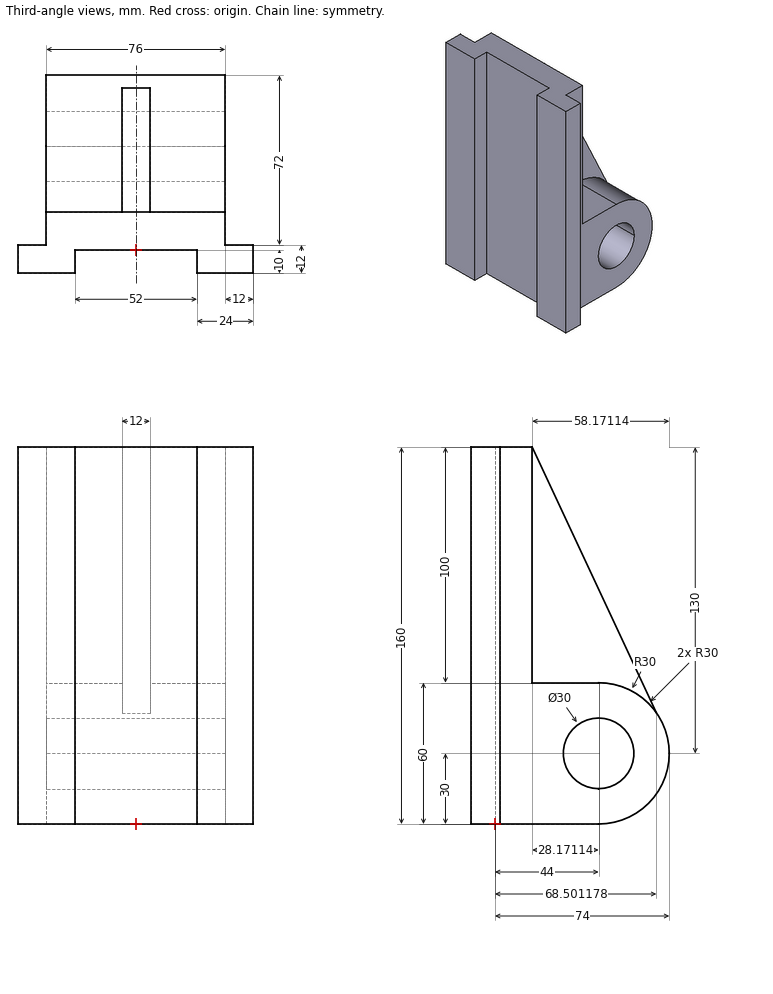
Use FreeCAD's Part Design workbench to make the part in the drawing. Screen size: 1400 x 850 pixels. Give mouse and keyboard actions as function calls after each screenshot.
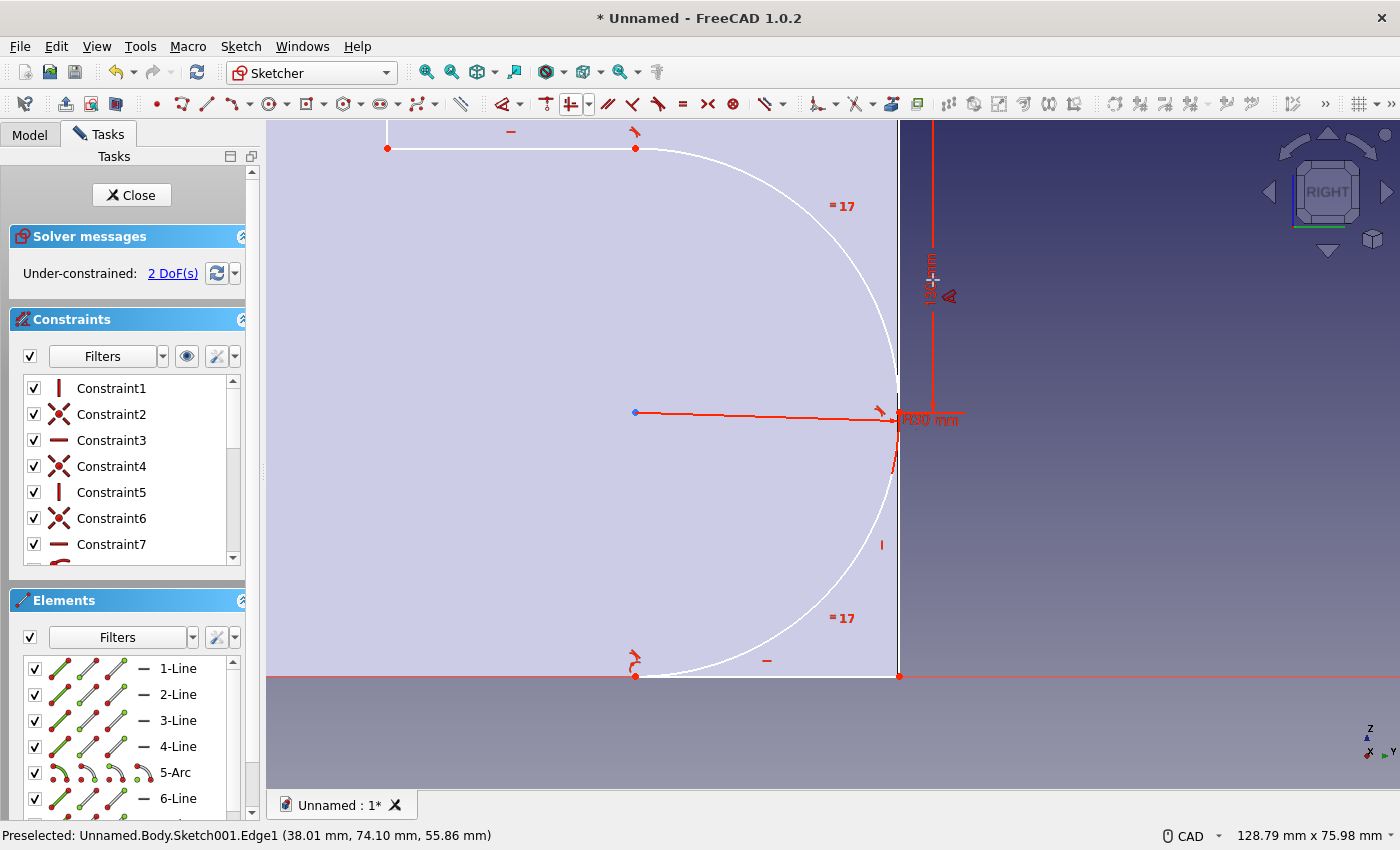
click(899, 413)
click(597, 711)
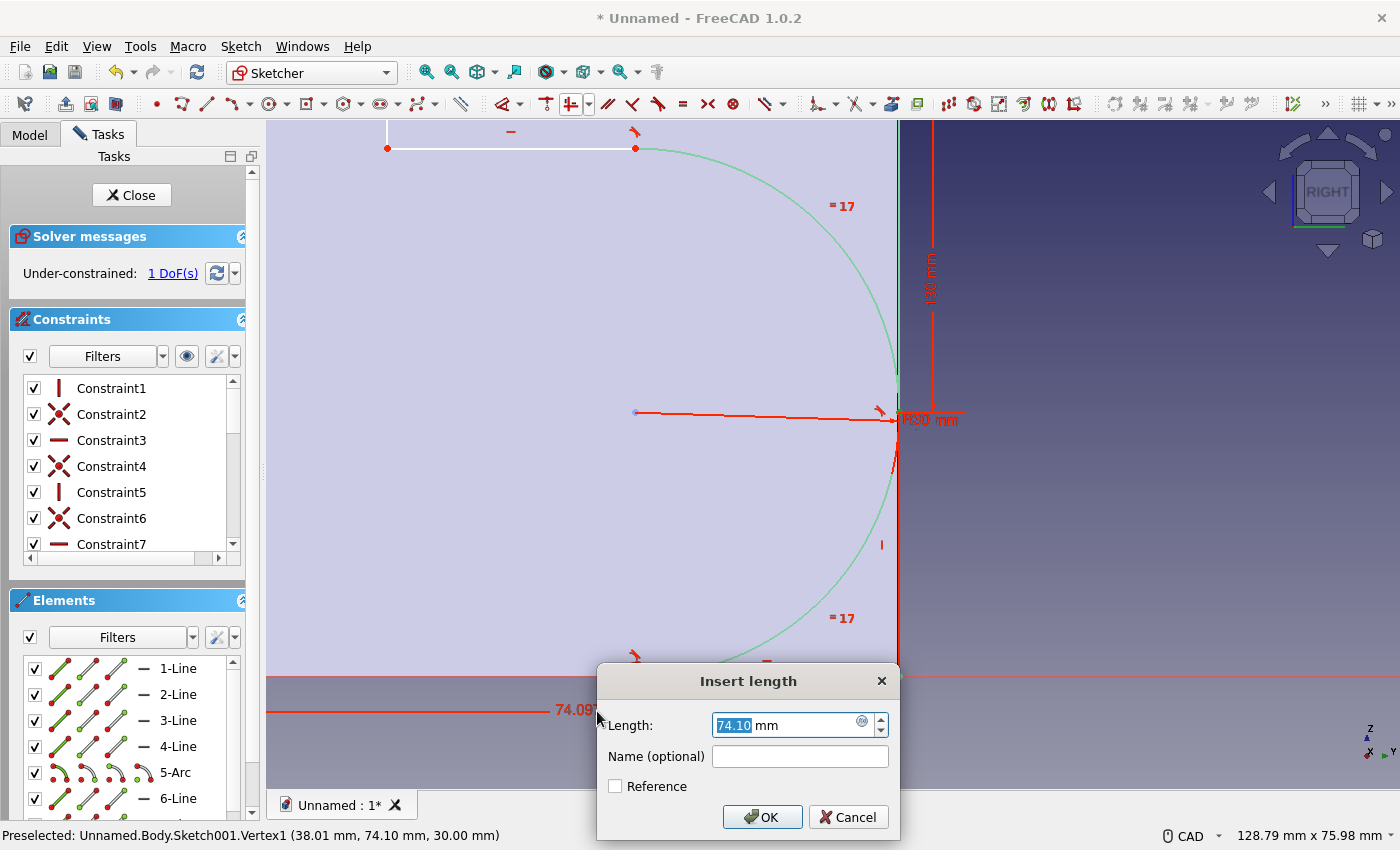
text(74)
key(Return)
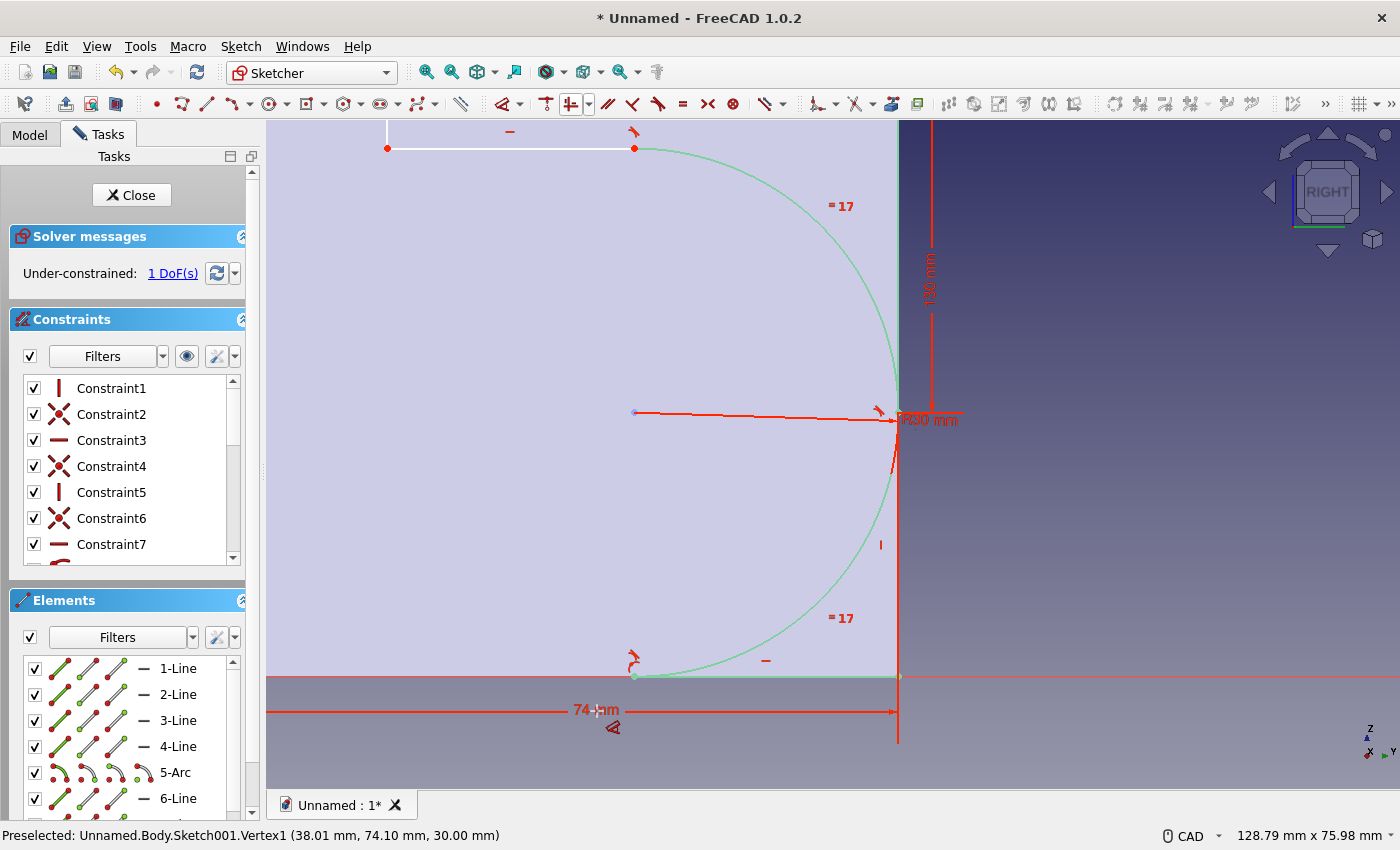
scroll(847, 662, down, 6)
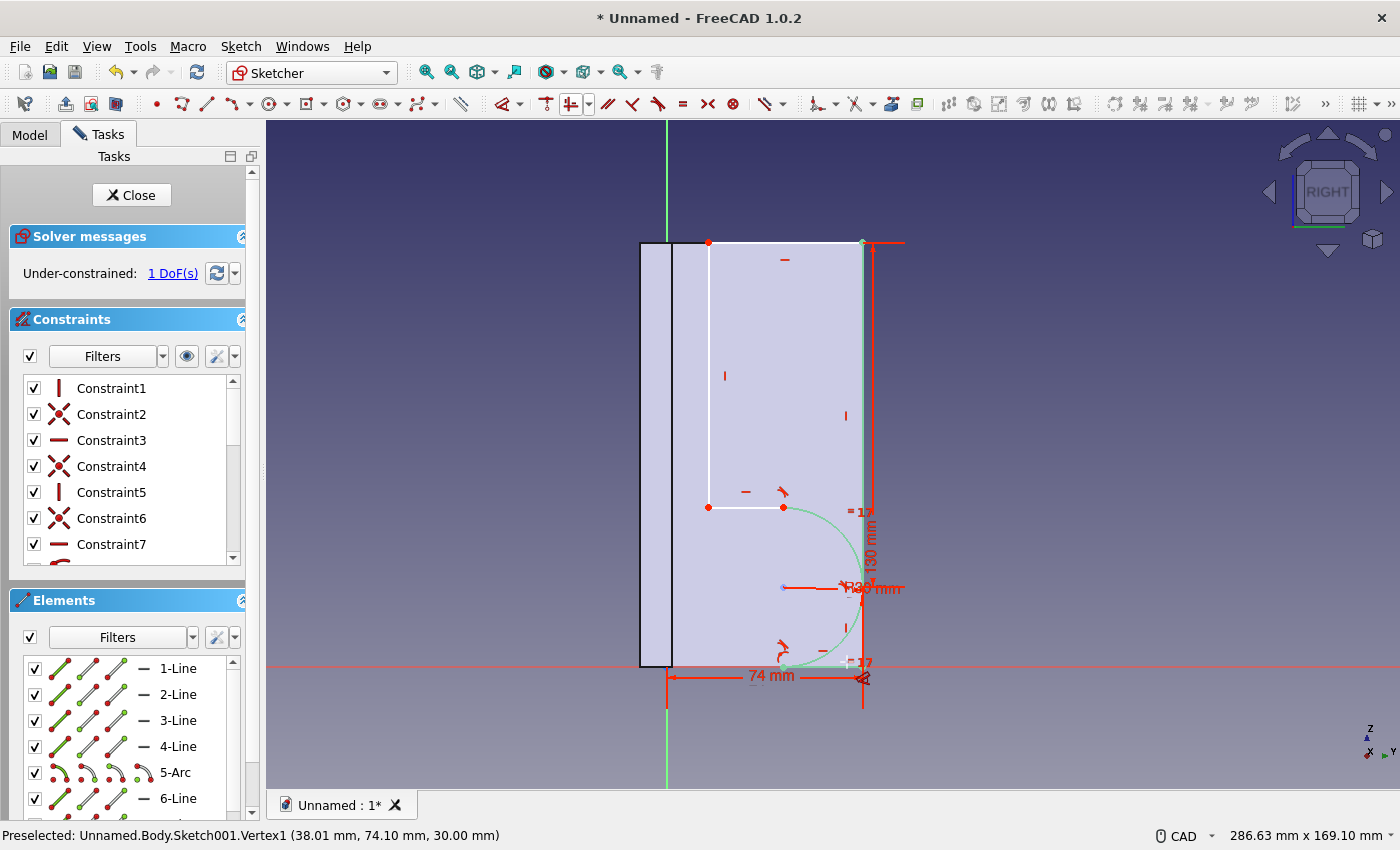
click(817, 243)
click(786, 209)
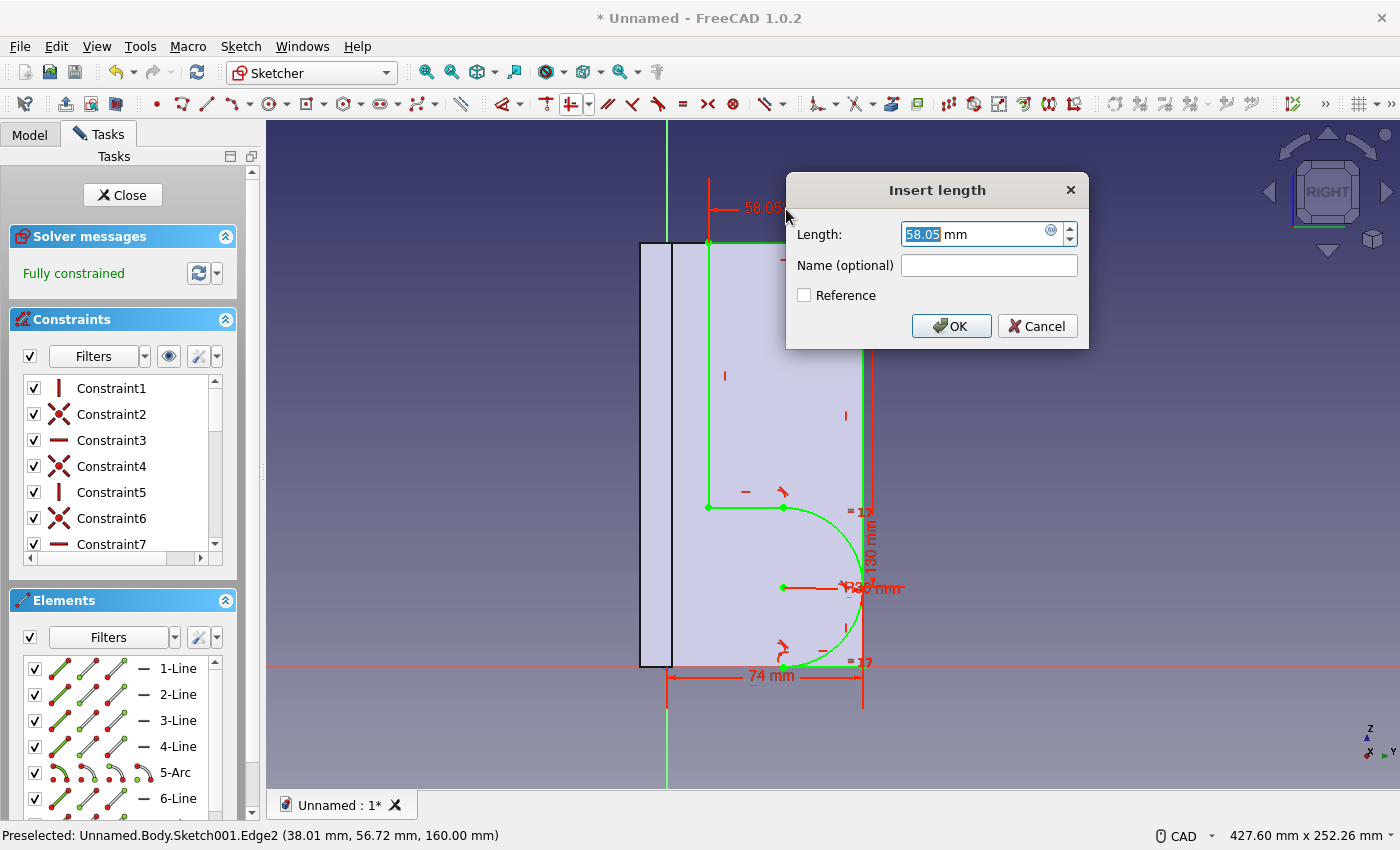
text(58.17114)
key(Return)
key(Escape)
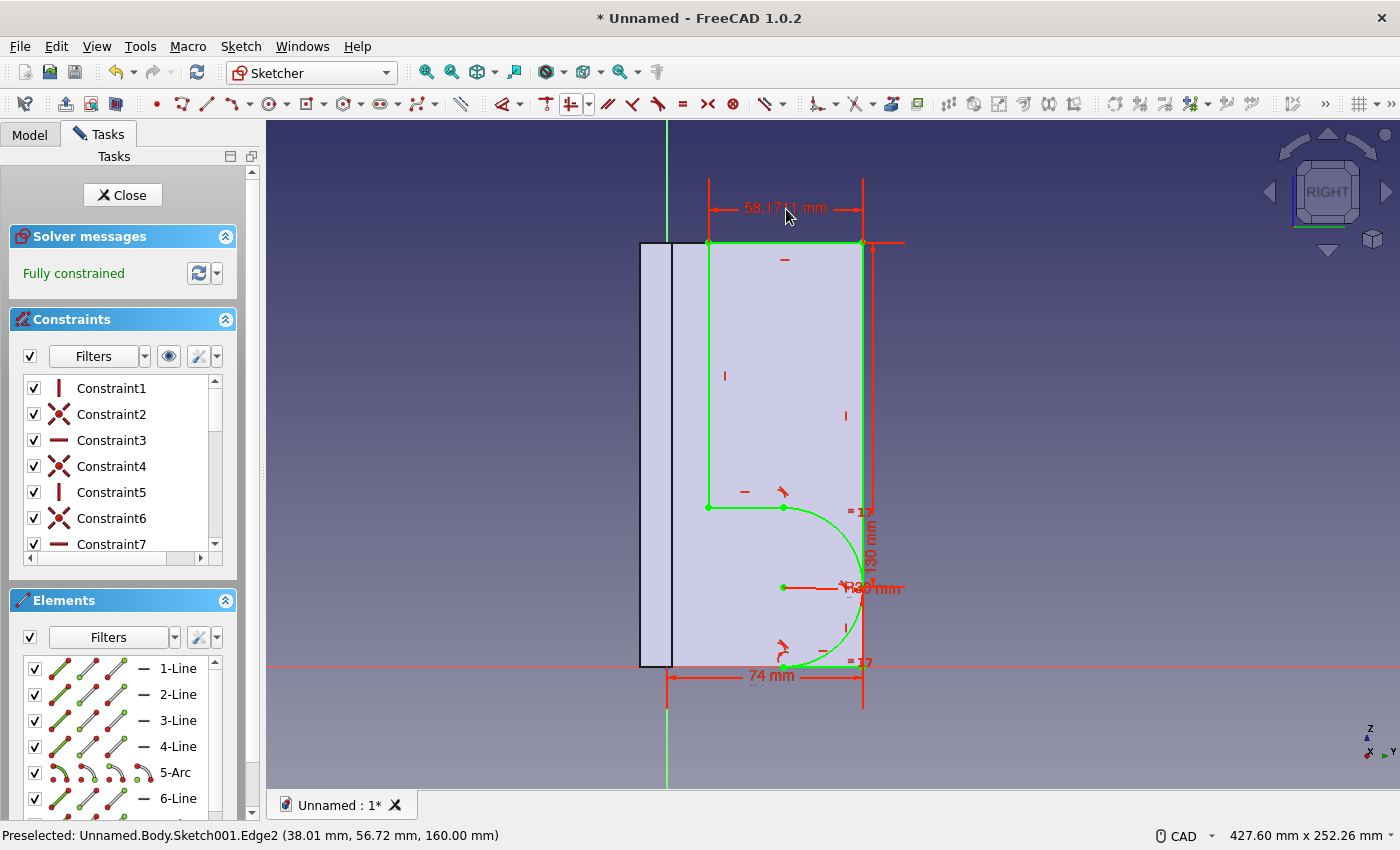
click(123, 195)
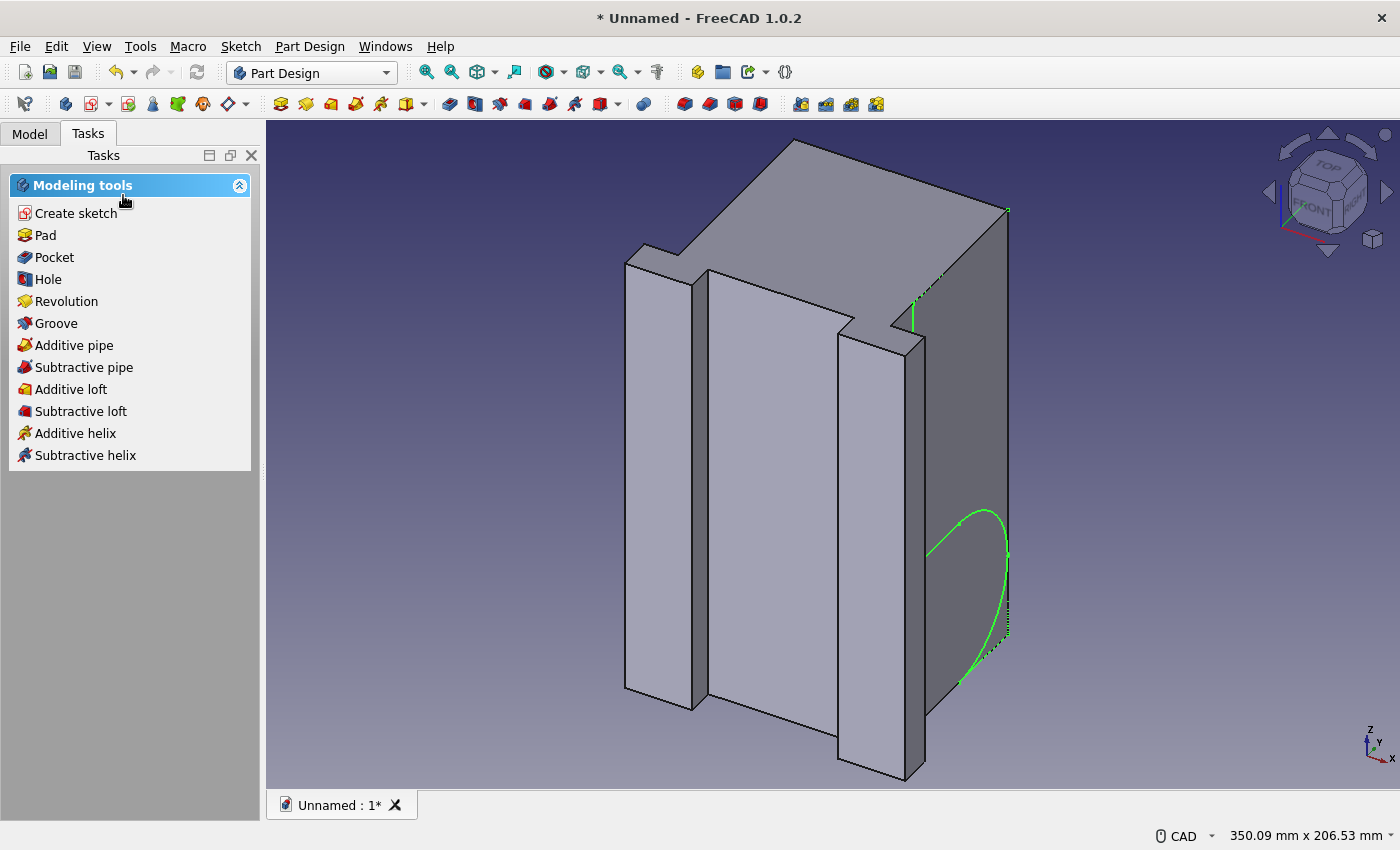
click(450, 104)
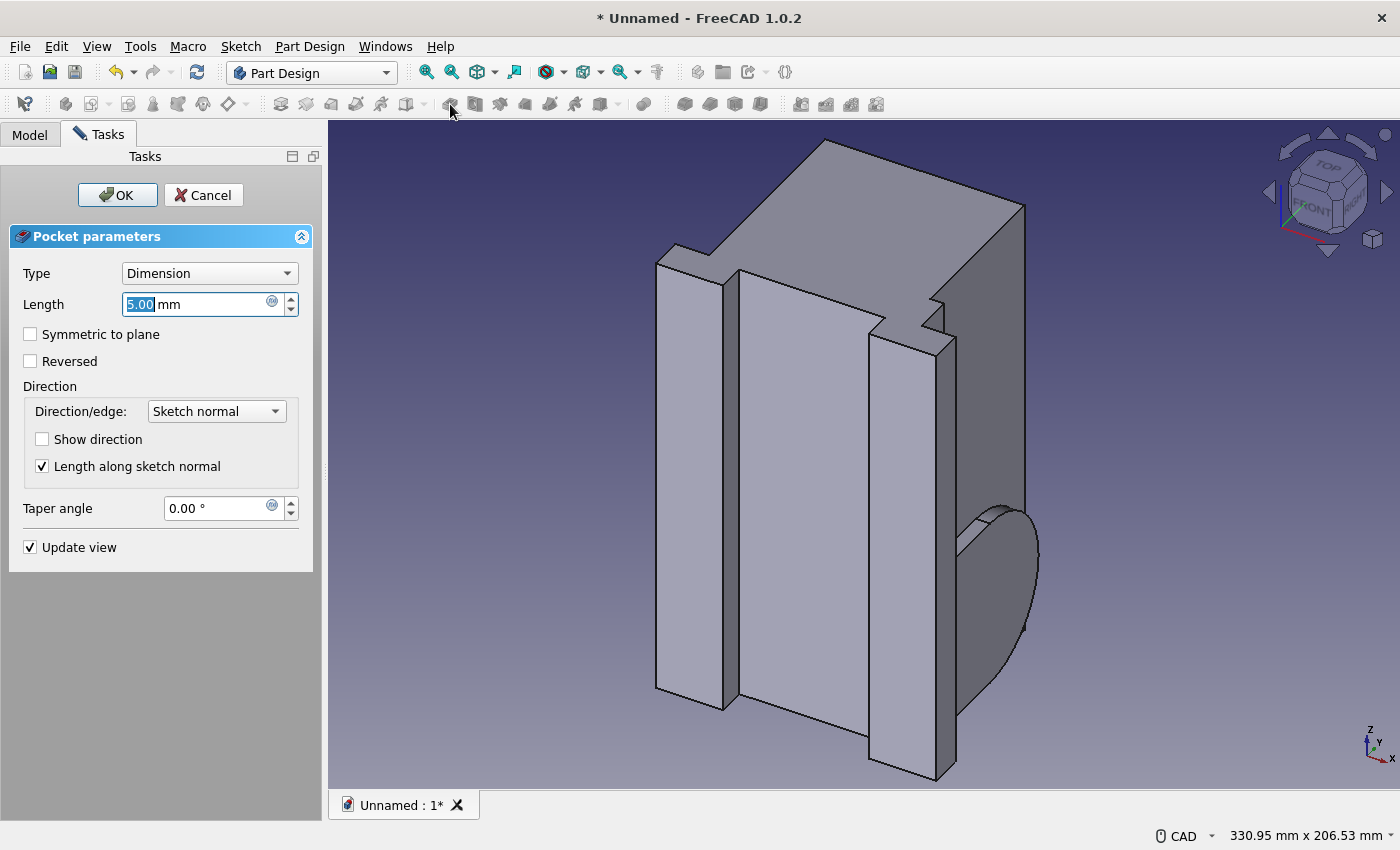
click(210, 274)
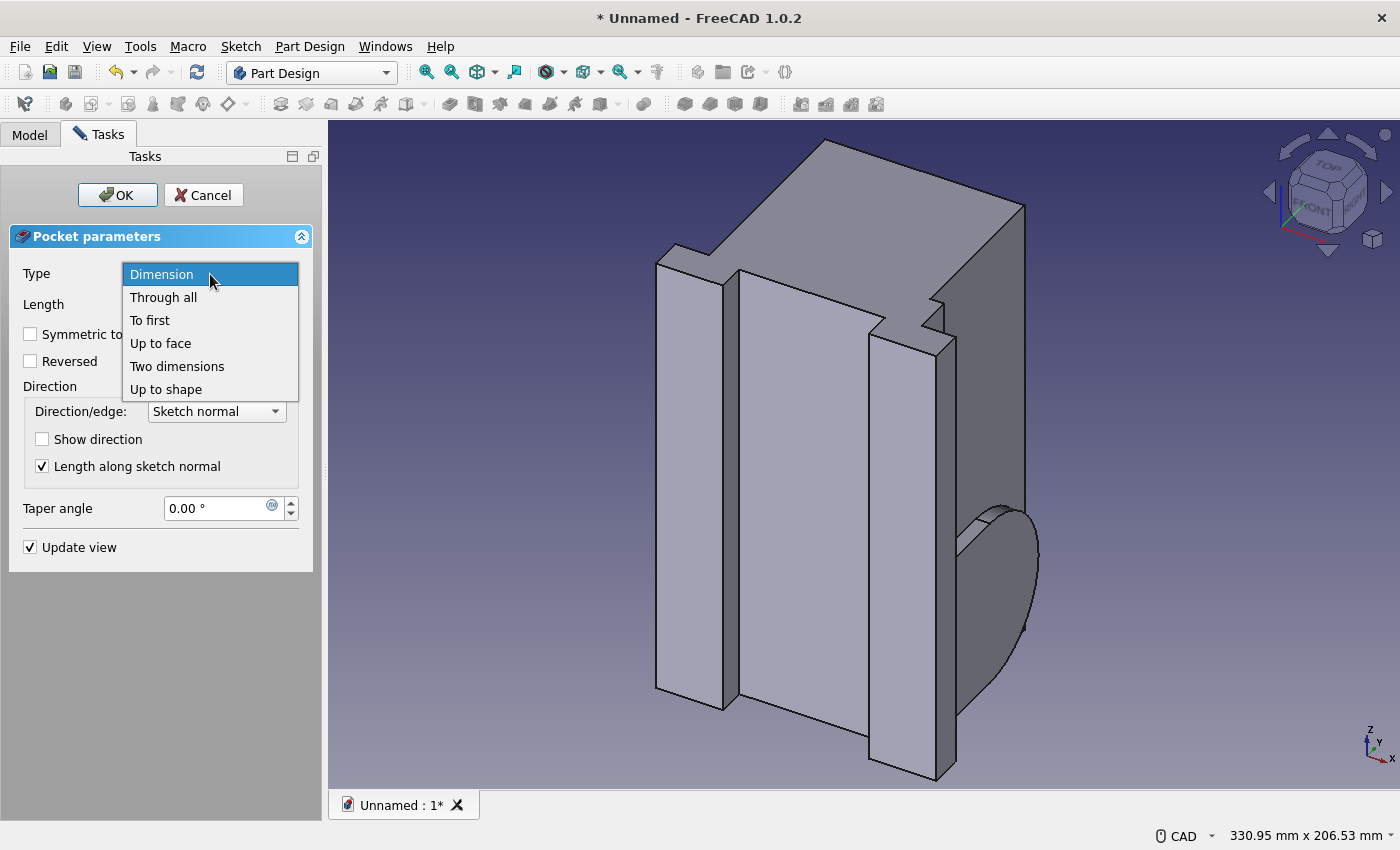
click(208, 298)